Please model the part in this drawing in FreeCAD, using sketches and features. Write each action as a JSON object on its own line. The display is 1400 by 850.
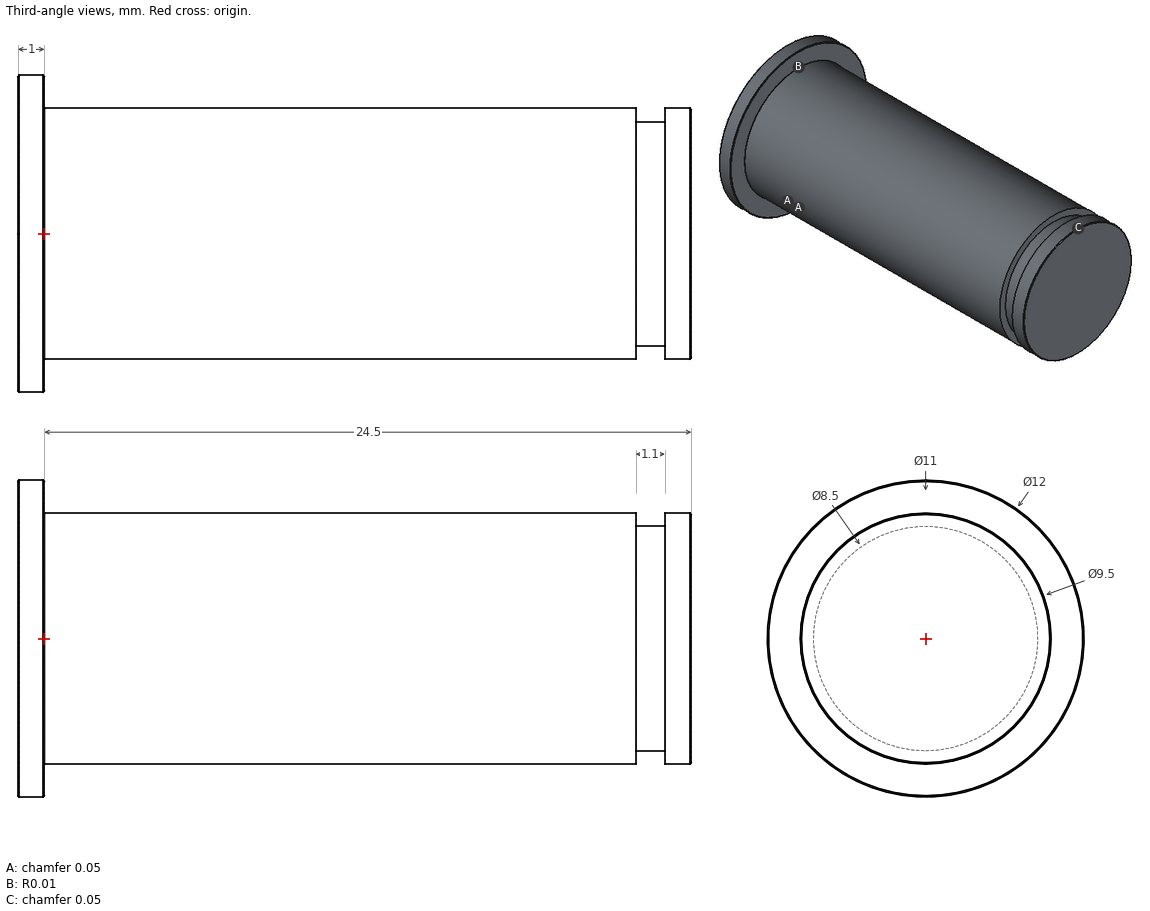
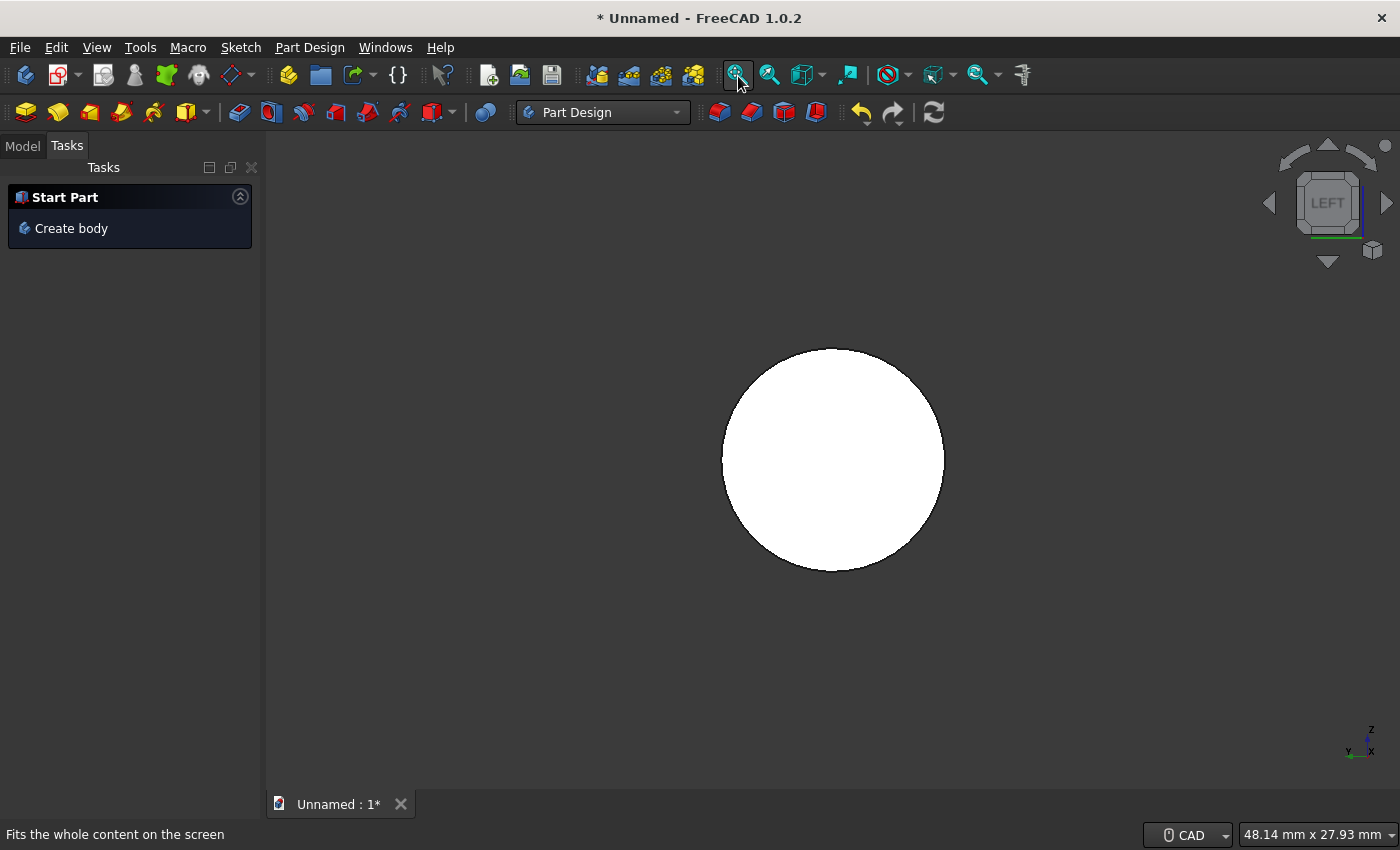
{"action": "key", "text": "v f"}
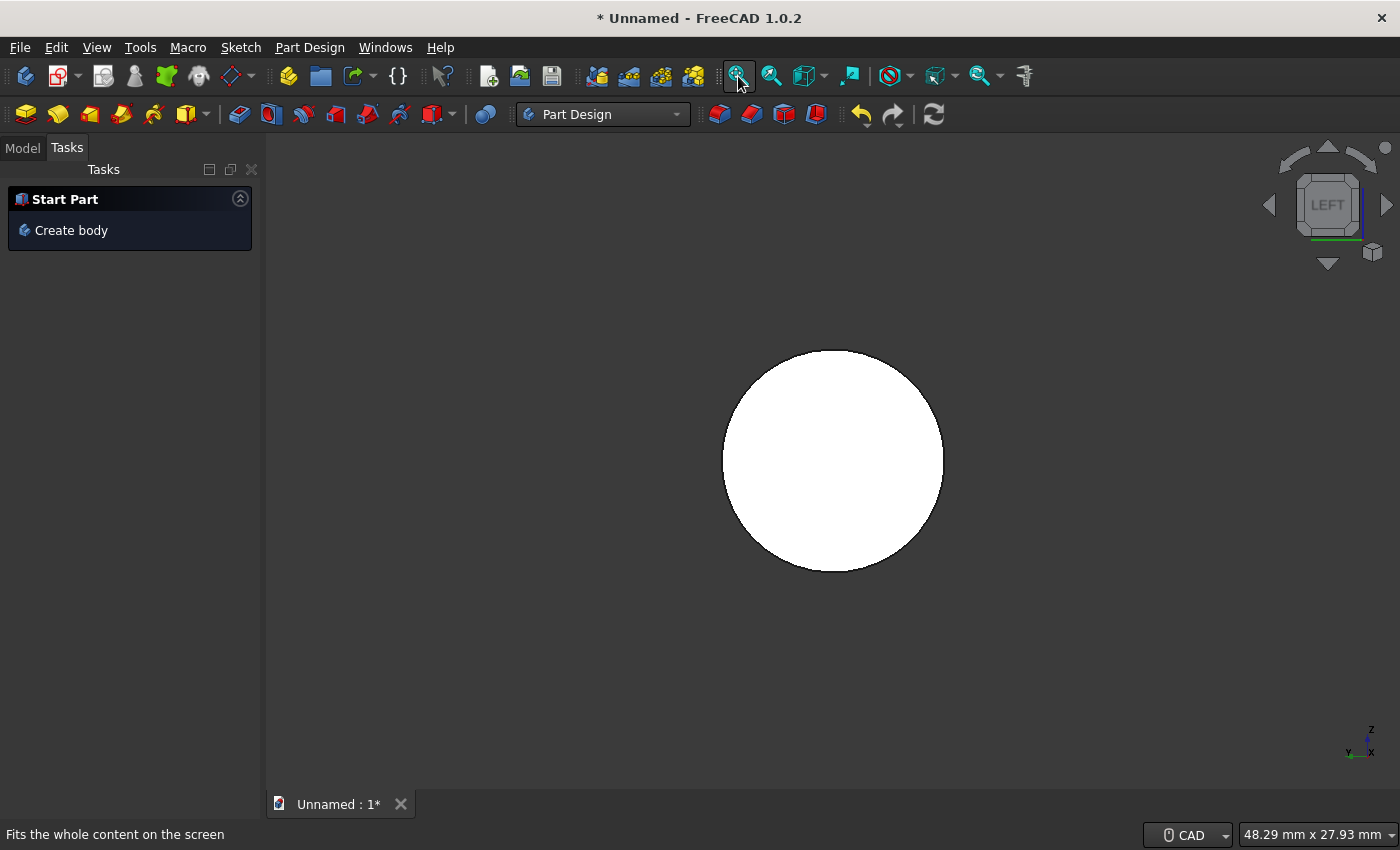
{"action": "left_click", "coordinate": [833, 460]}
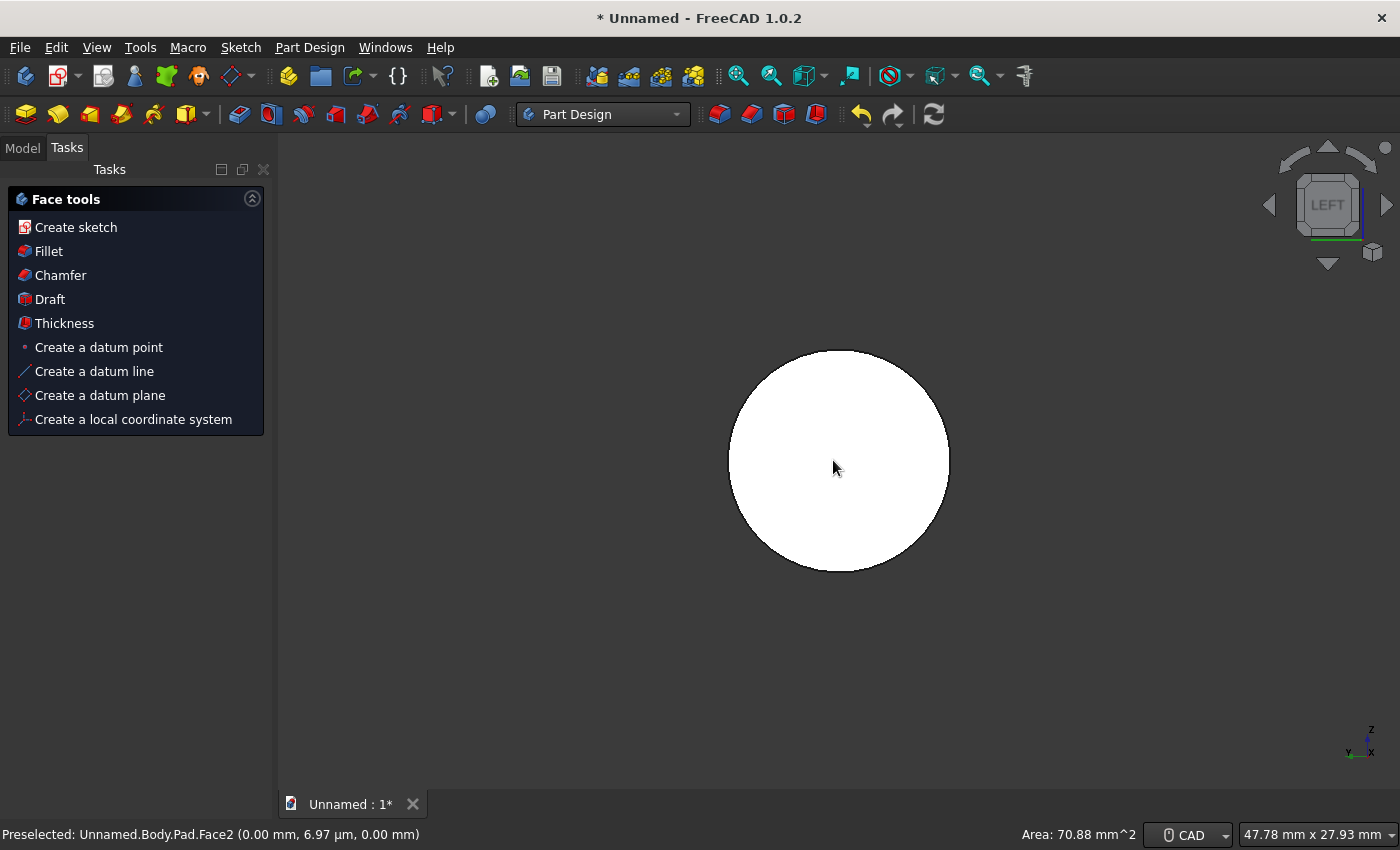
{"action": "left_click", "coordinate": [58, 76]}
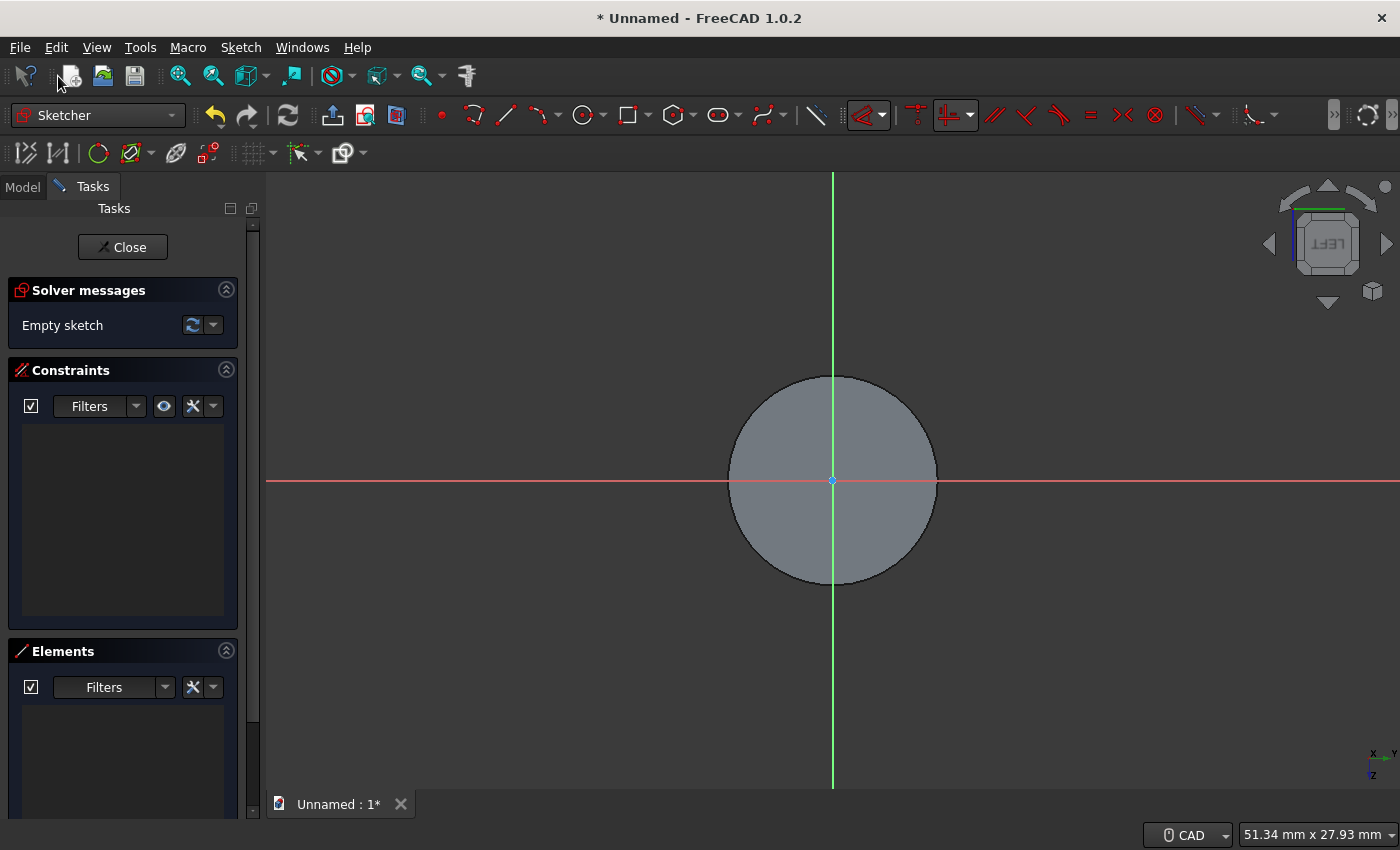
{"action": "scroll", "coordinate": [972, 480], "scroll_direction": "up", "scroll_amount": 2}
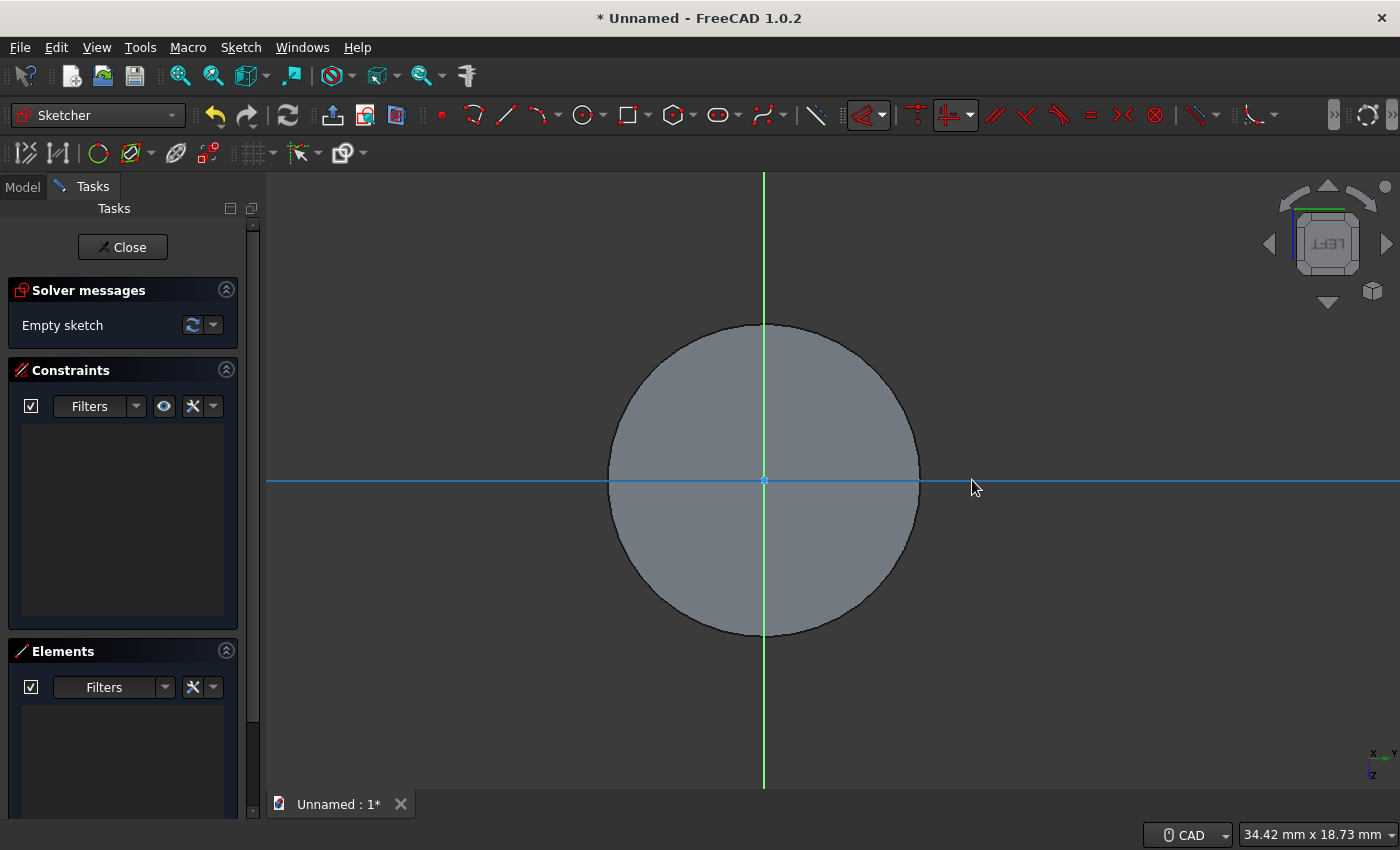
{"action": "left_click", "coordinate": [584, 116]}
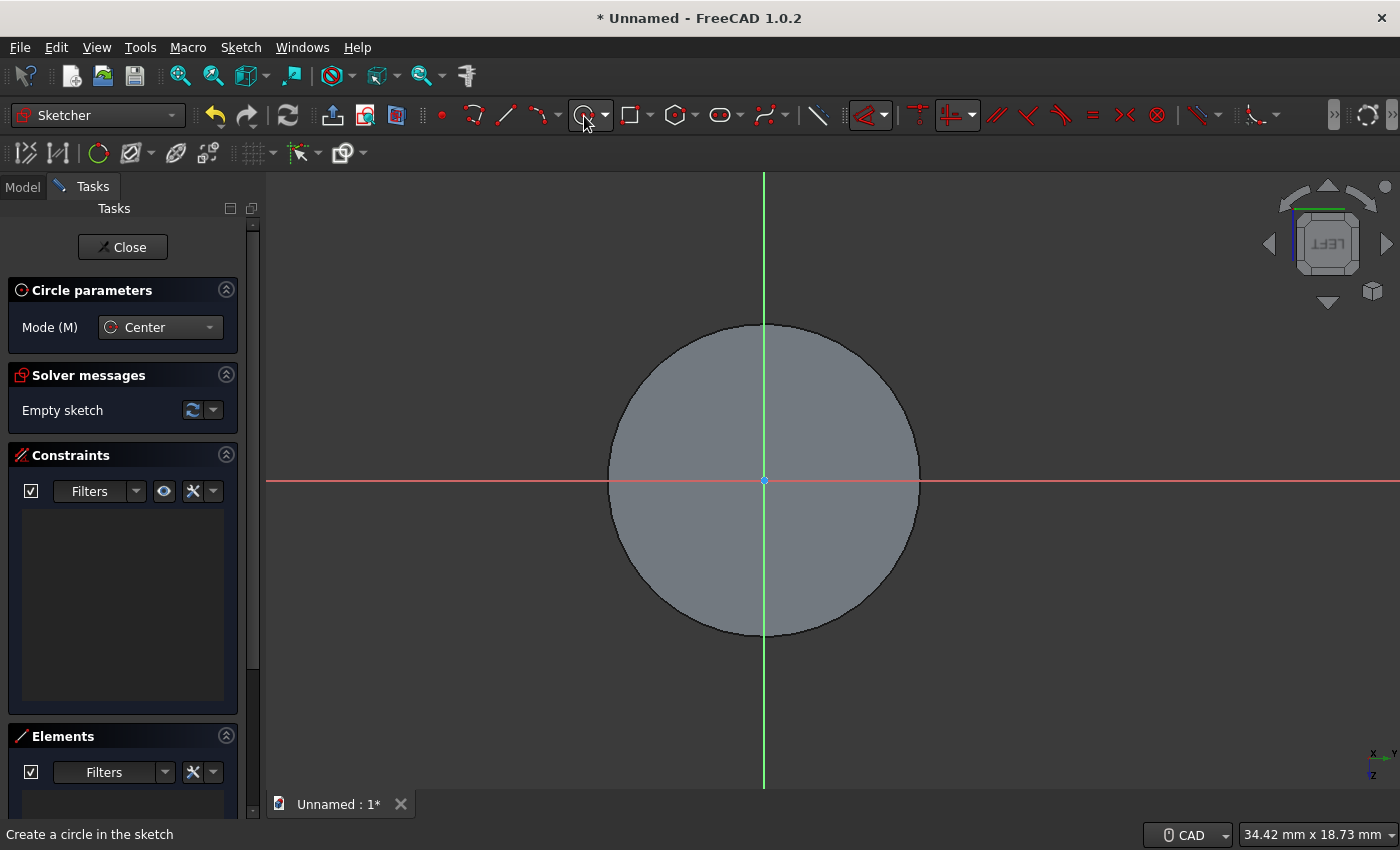
{"action": "left_click", "coordinate": [764, 480]}
{"action": "left_click", "coordinate": [904, 341]}
{"action": "key", "text": "Escape"}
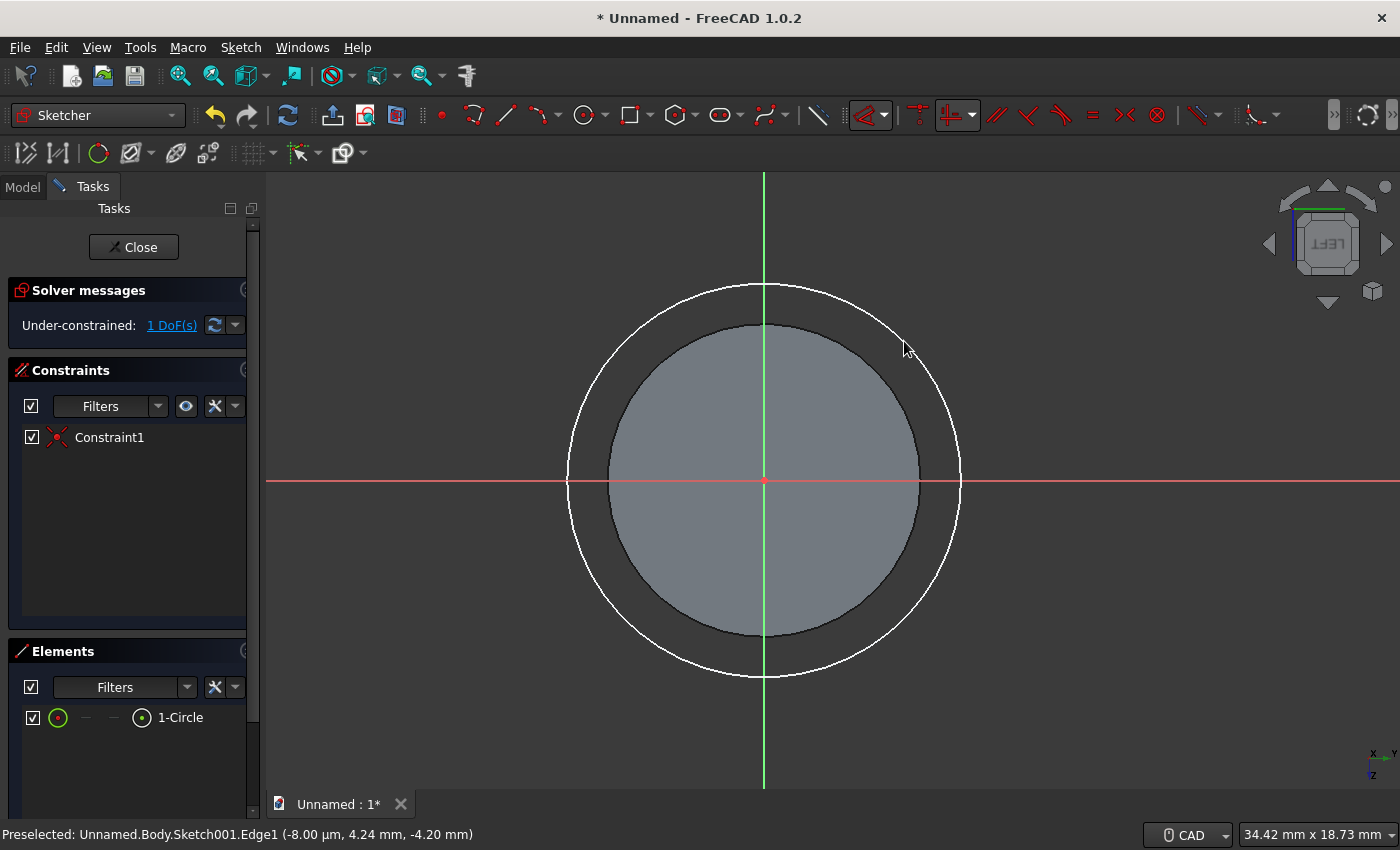
{"action": "key", "text": "d"}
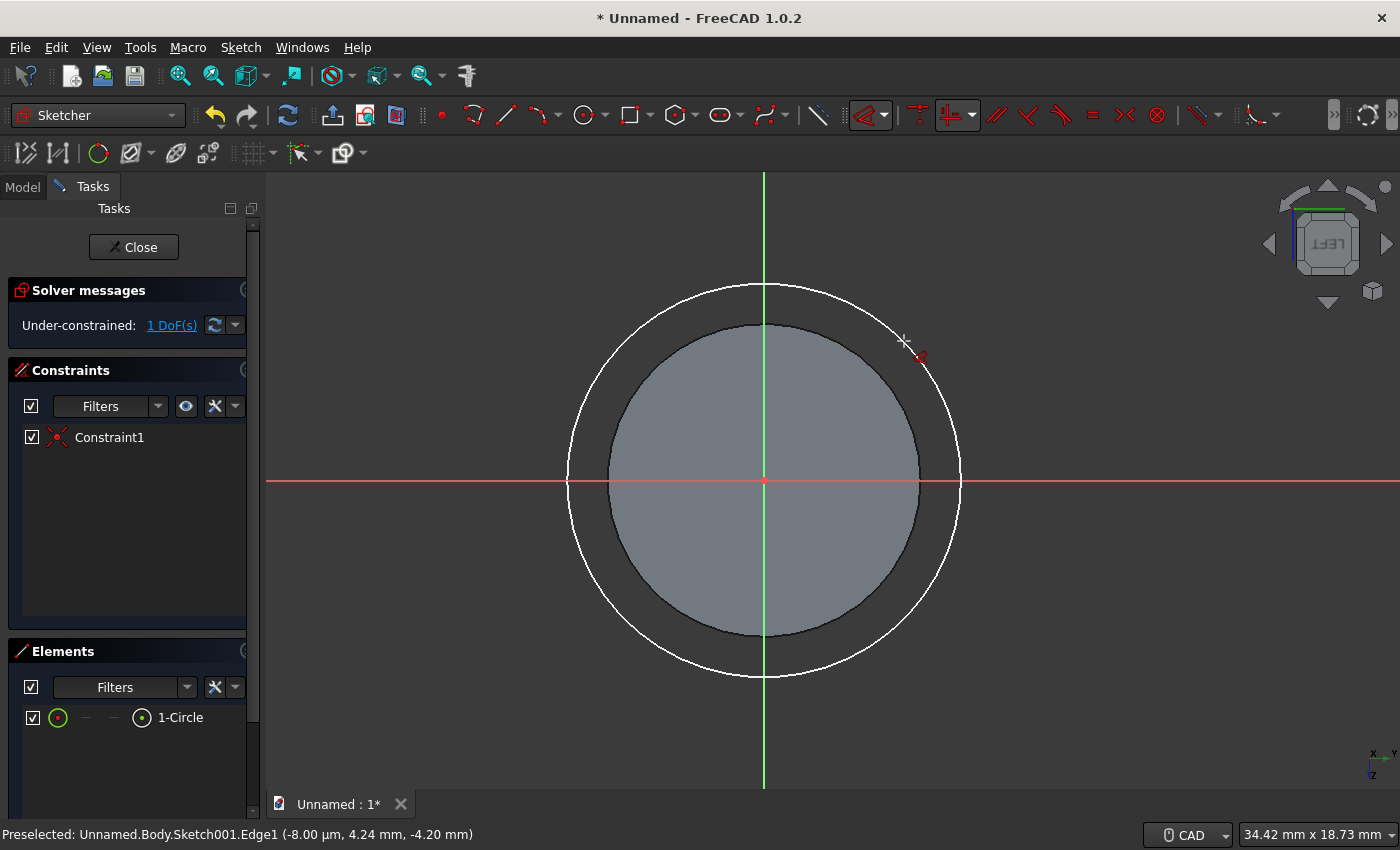
{"action": "left_click", "coordinate": [903, 341]}
{"action": "left_click", "coordinate": [926, 318]}